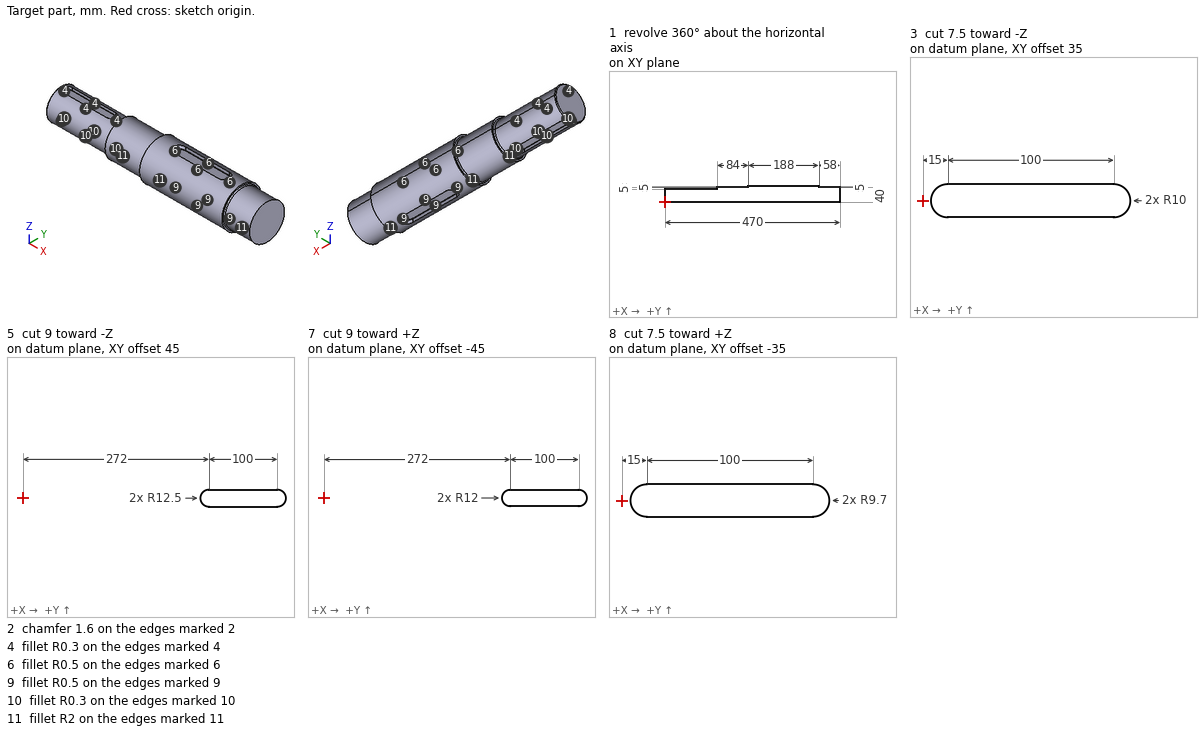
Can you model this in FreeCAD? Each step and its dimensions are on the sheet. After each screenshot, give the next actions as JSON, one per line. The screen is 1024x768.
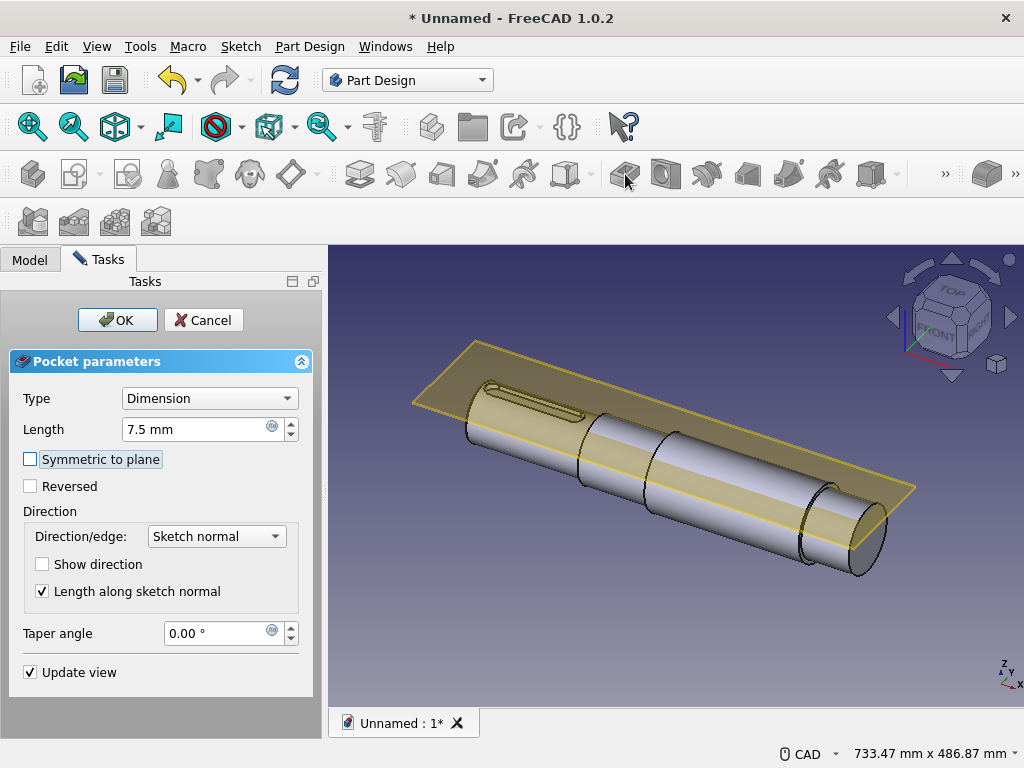
{"action": "left_click", "coordinate": [118, 320]}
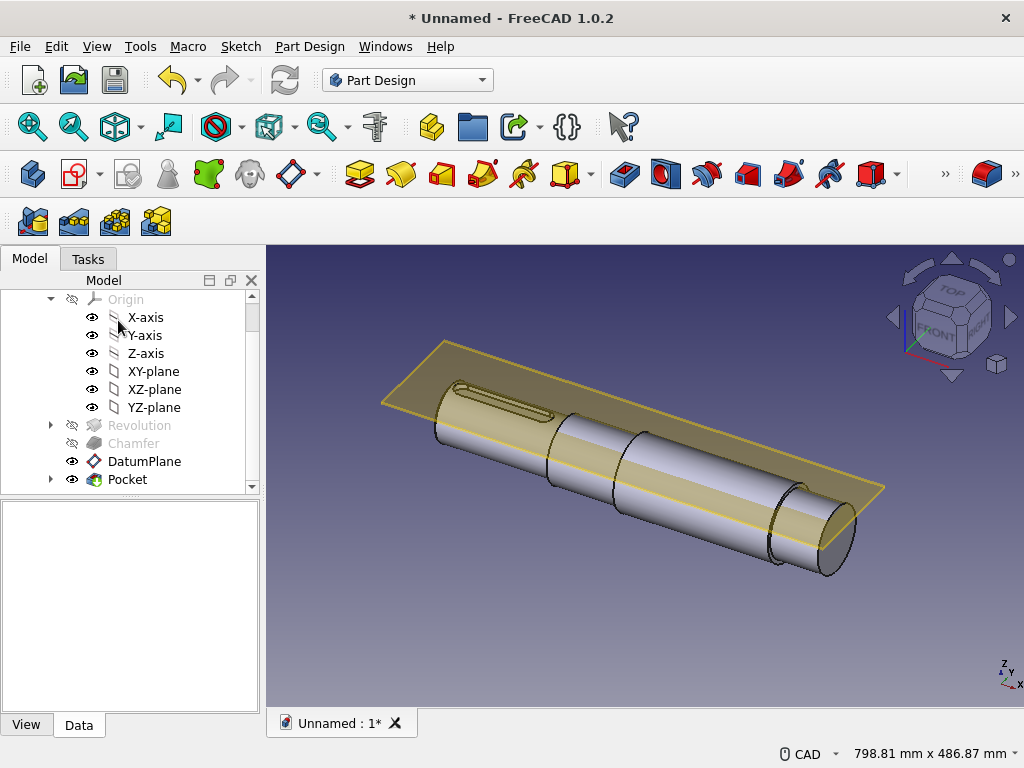
{"action": "left_click", "coordinate": [117, 461]}
{"action": "key", "text": "space"}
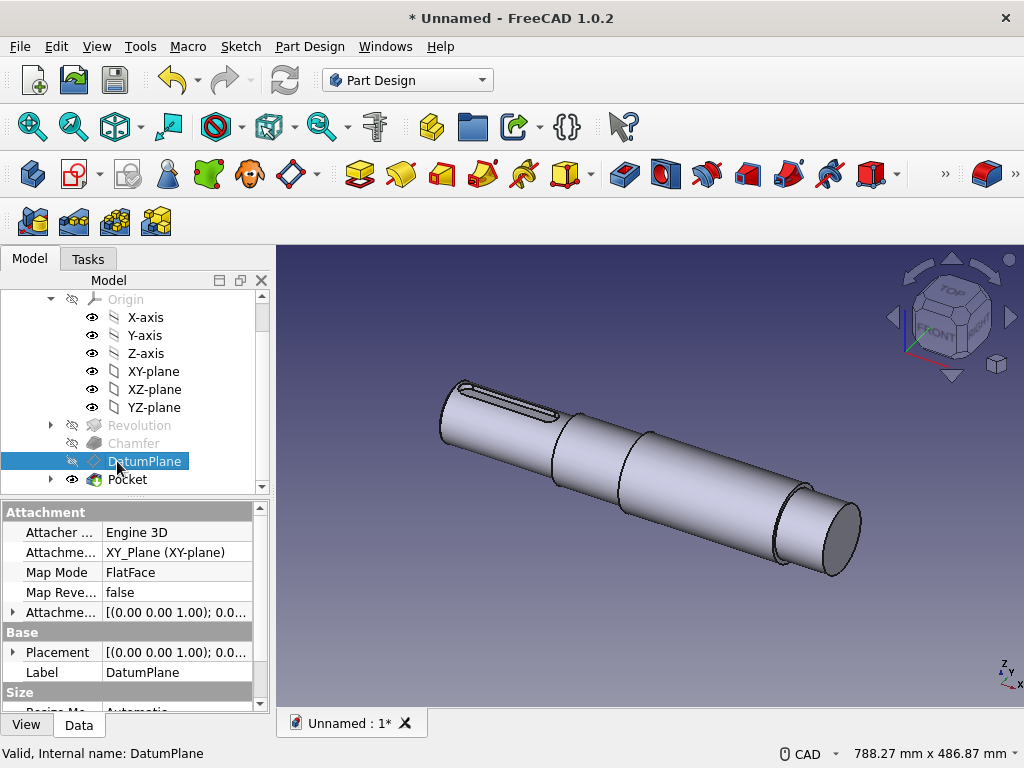
{"action": "key", "text": "0"}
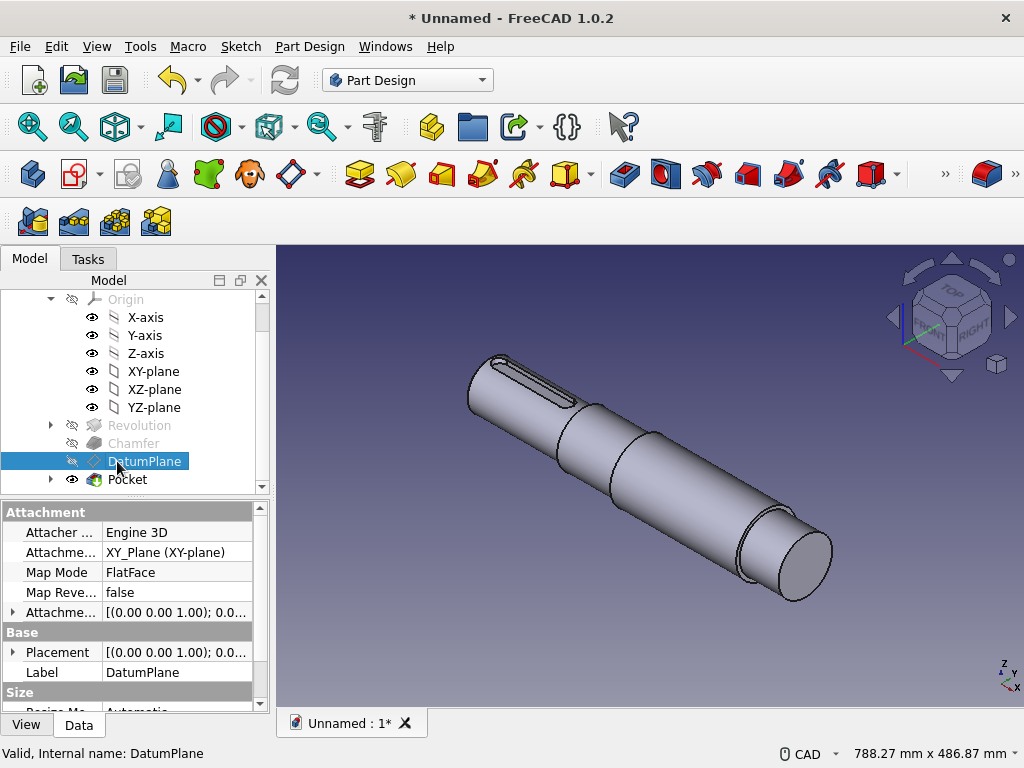
{"action": "key", "text": "2"}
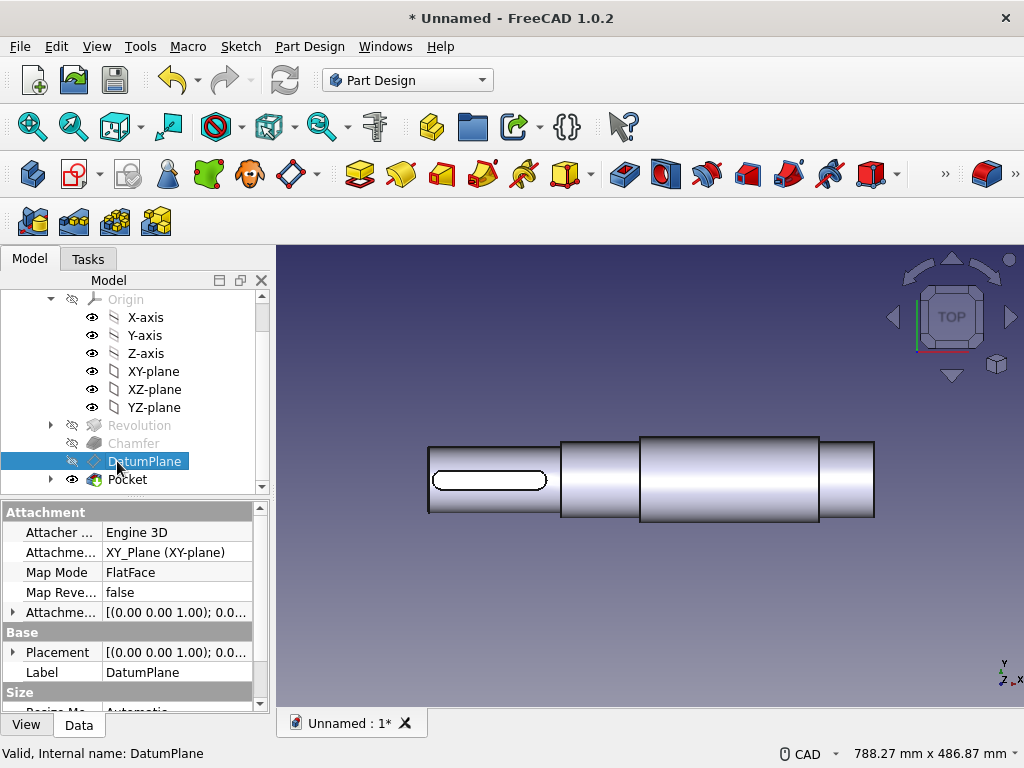
{"action": "left_click", "coordinate": [522, 479]}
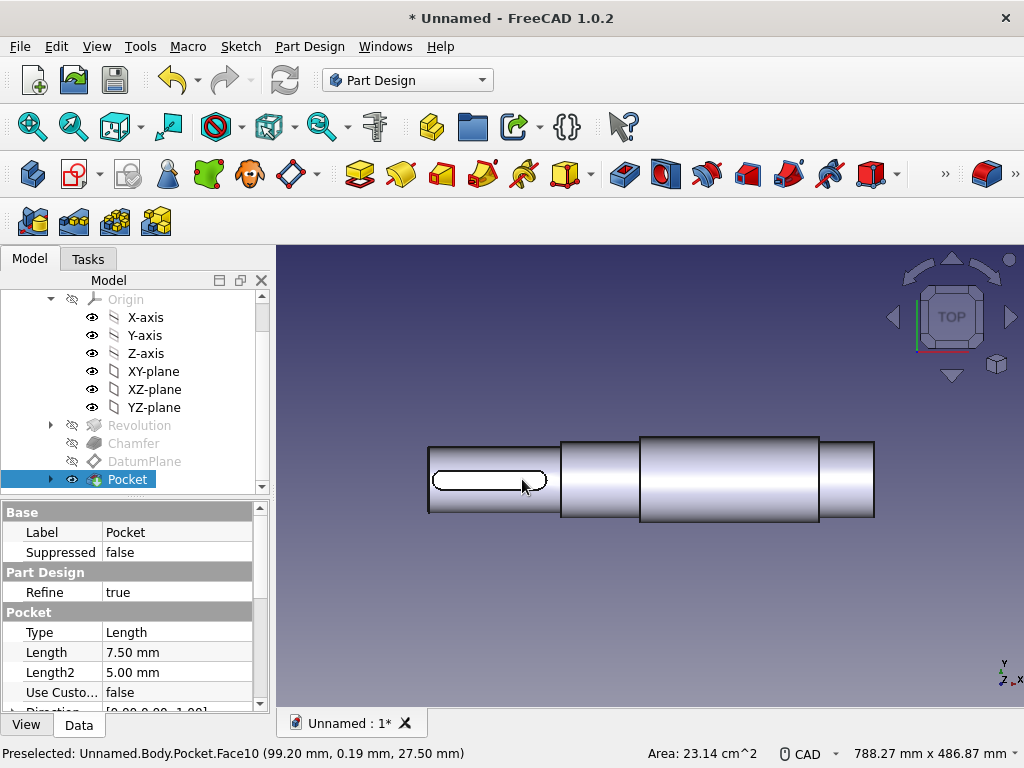
{"action": "left_click", "coordinate": [987, 174]}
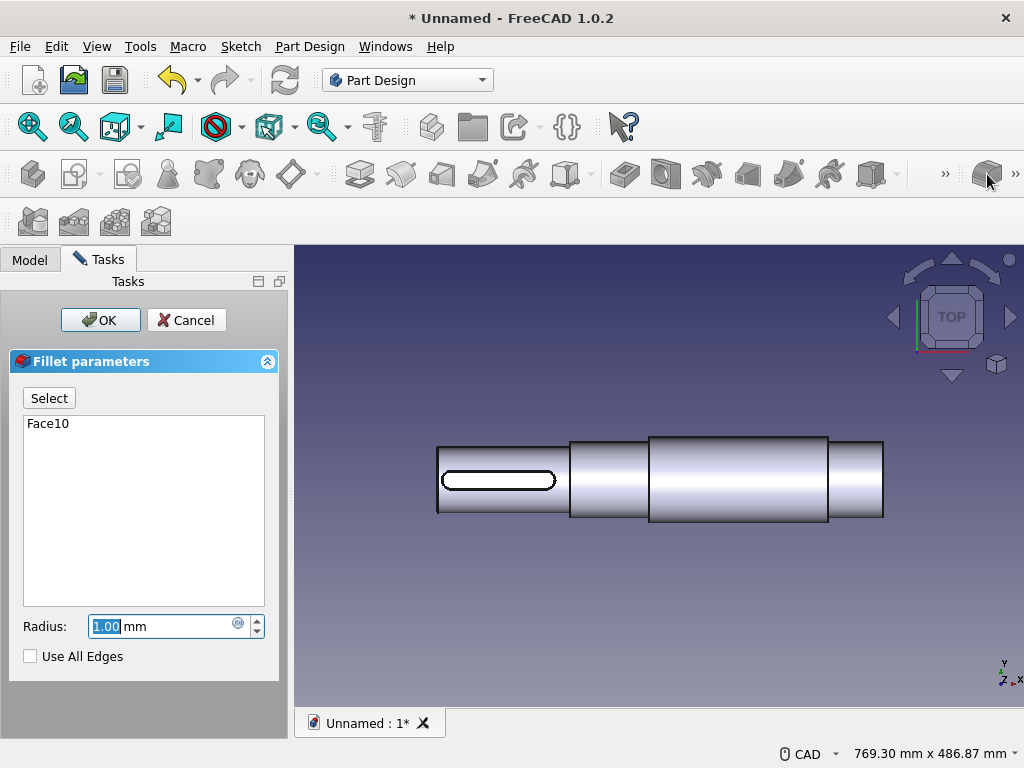
{"action": "type", "text": "0.3"}
{"action": "key", "text": "Tab"}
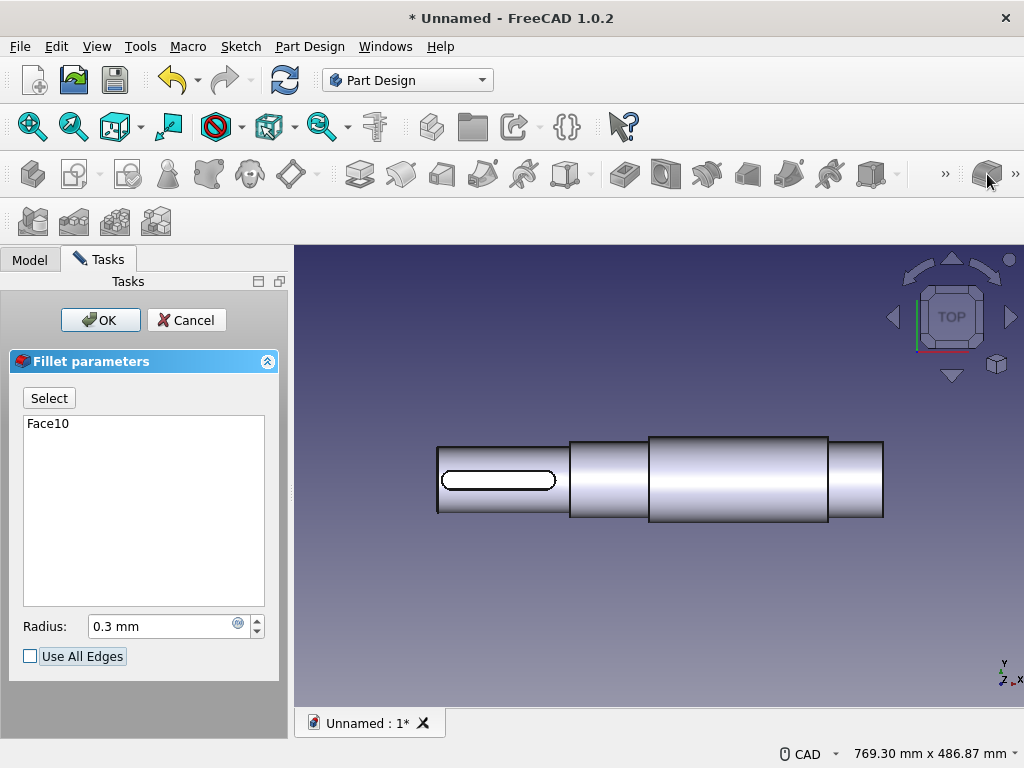
{"action": "left_click", "coordinate": [101, 320]}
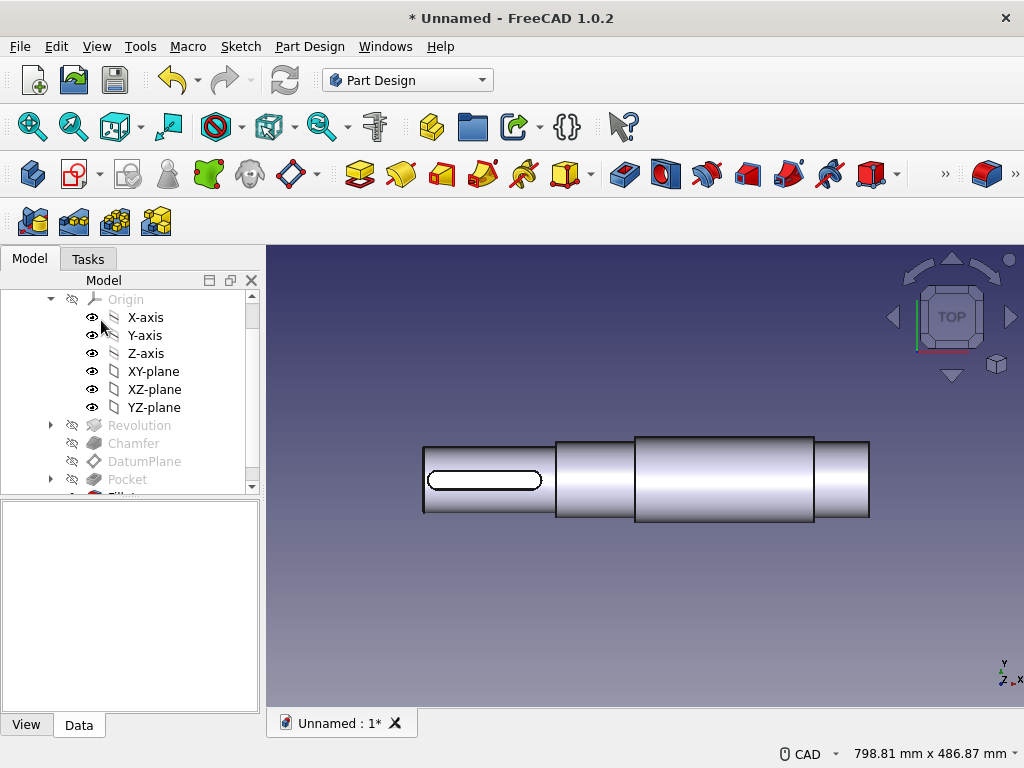
{"action": "left_click", "coordinate": [137, 371]}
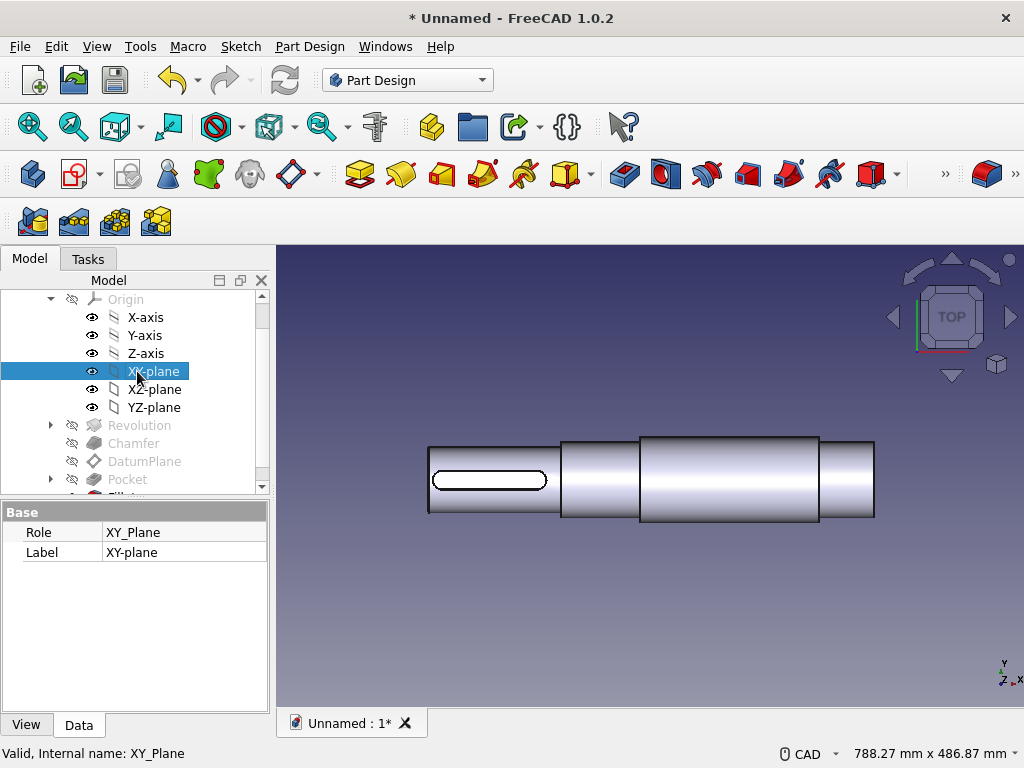
{"action": "left_click", "coordinate": [290, 174]}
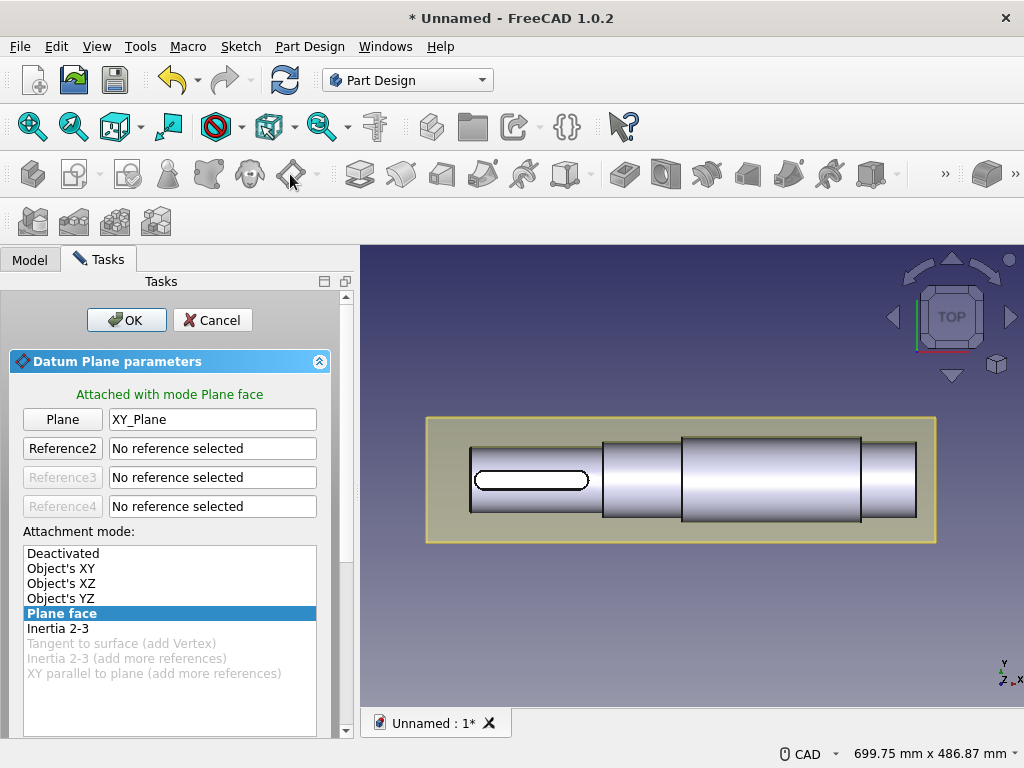
{"action": "scroll", "coordinate": [346, 514], "scroll_direction": "down", "scroll_amount": 4}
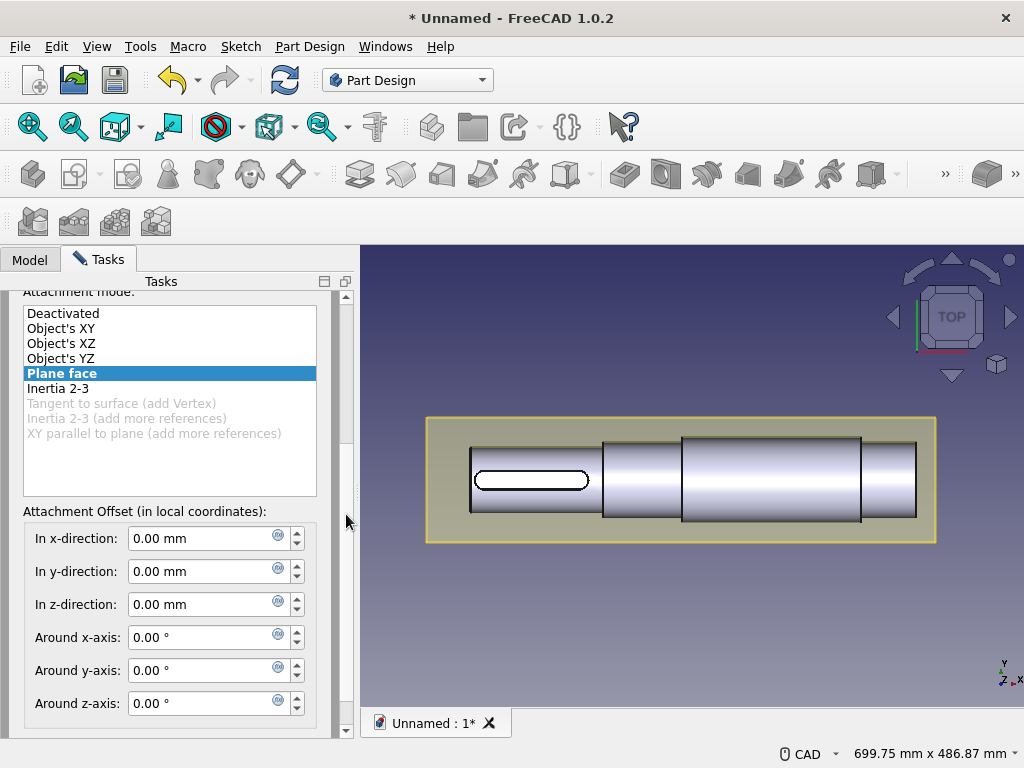
{"action": "triple_click", "coordinate": [210, 604]}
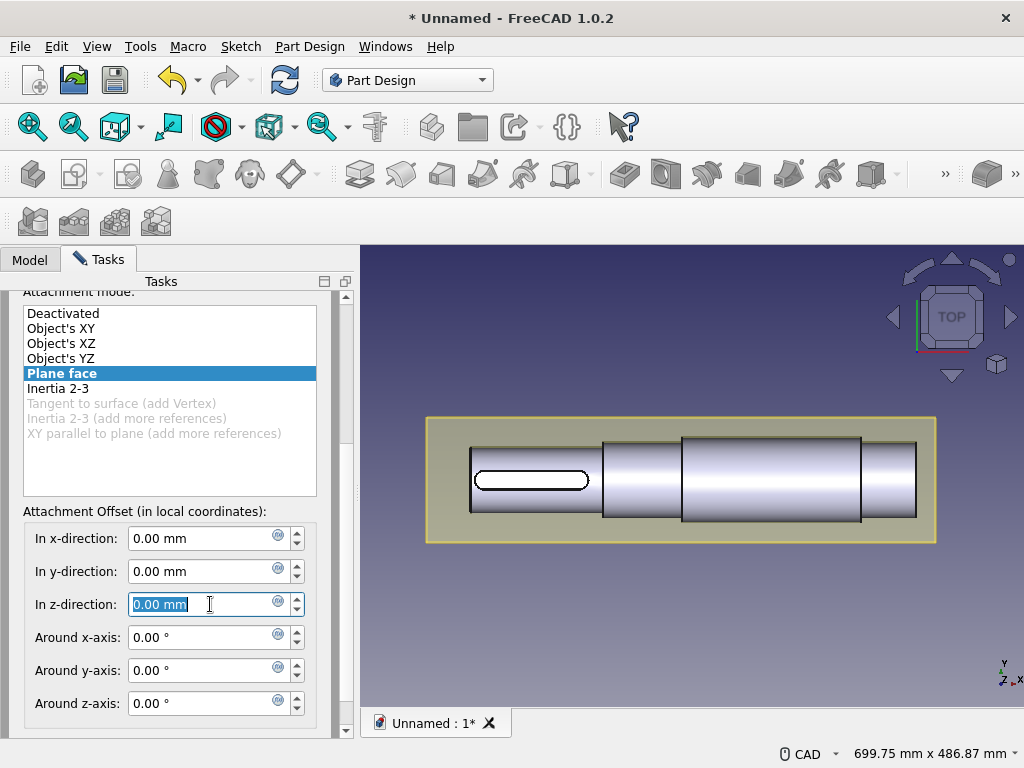
{"action": "type", "text": "45"}
{"action": "key", "text": "Tab"}